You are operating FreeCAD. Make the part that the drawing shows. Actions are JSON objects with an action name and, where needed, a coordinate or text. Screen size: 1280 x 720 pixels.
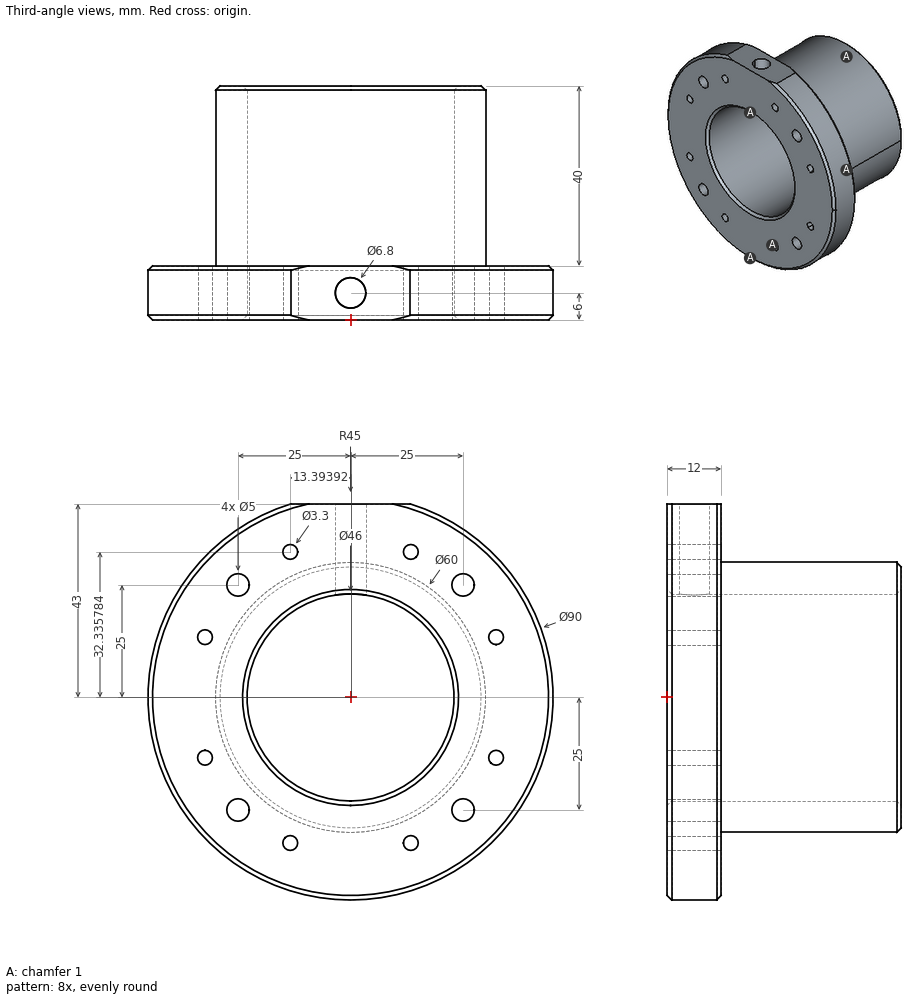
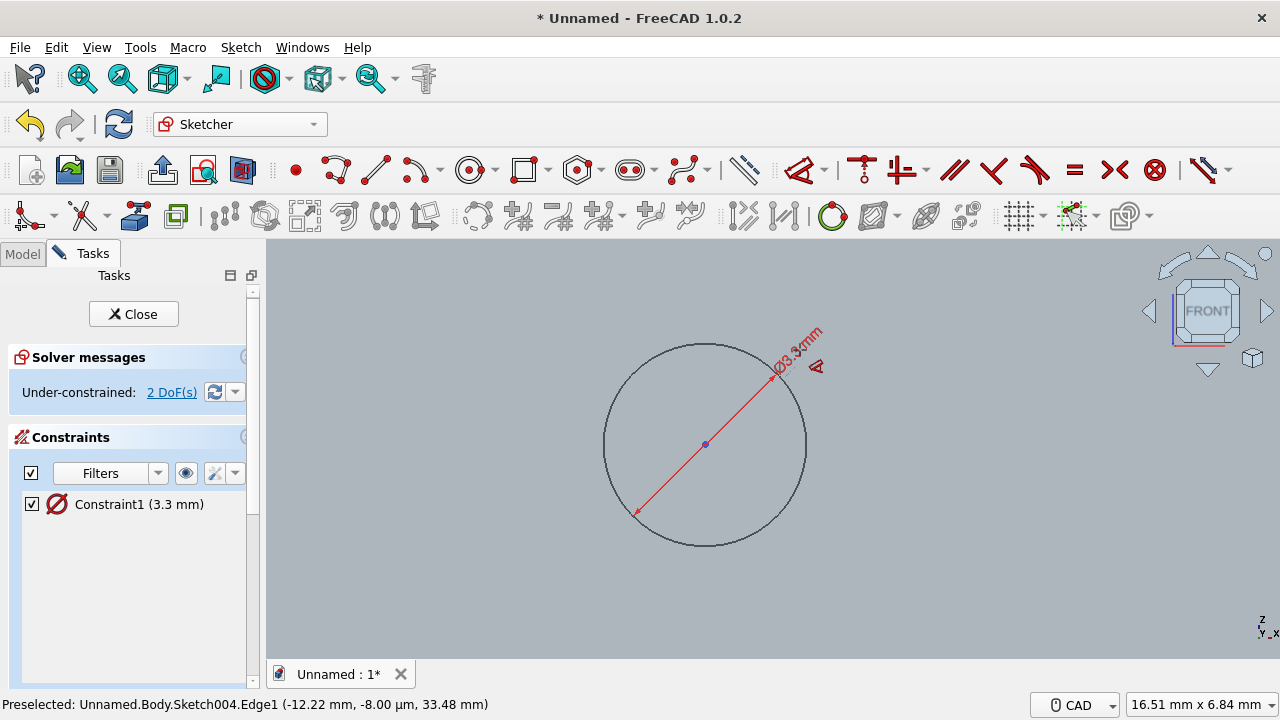
{"action": "left_click", "coordinate": [705, 445]}
{"action": "left_click", "coordinate": [910, 411]}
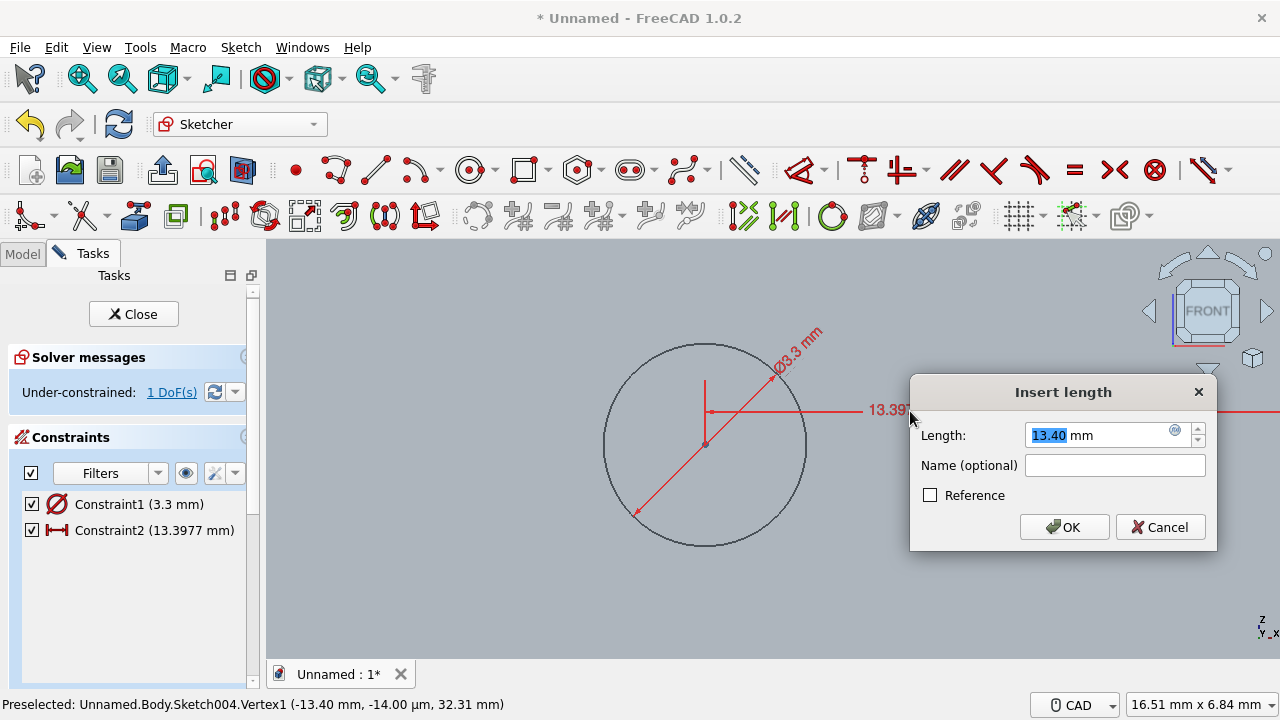
{"action": "type", "text": "13.39392"}
{"action": "key", "text": "Return"}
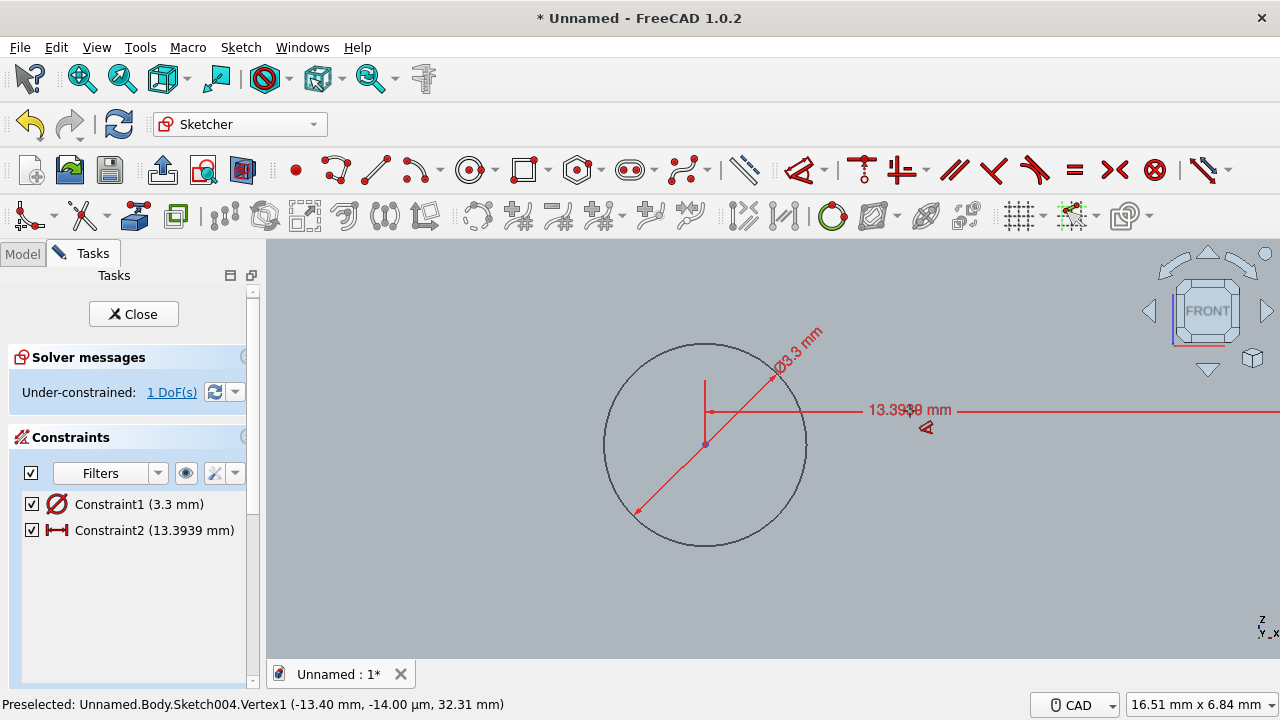
{"action": "left_click", "coordinate": [705, 445]}
{"action": "left_click", "coordinate": [671, 495]}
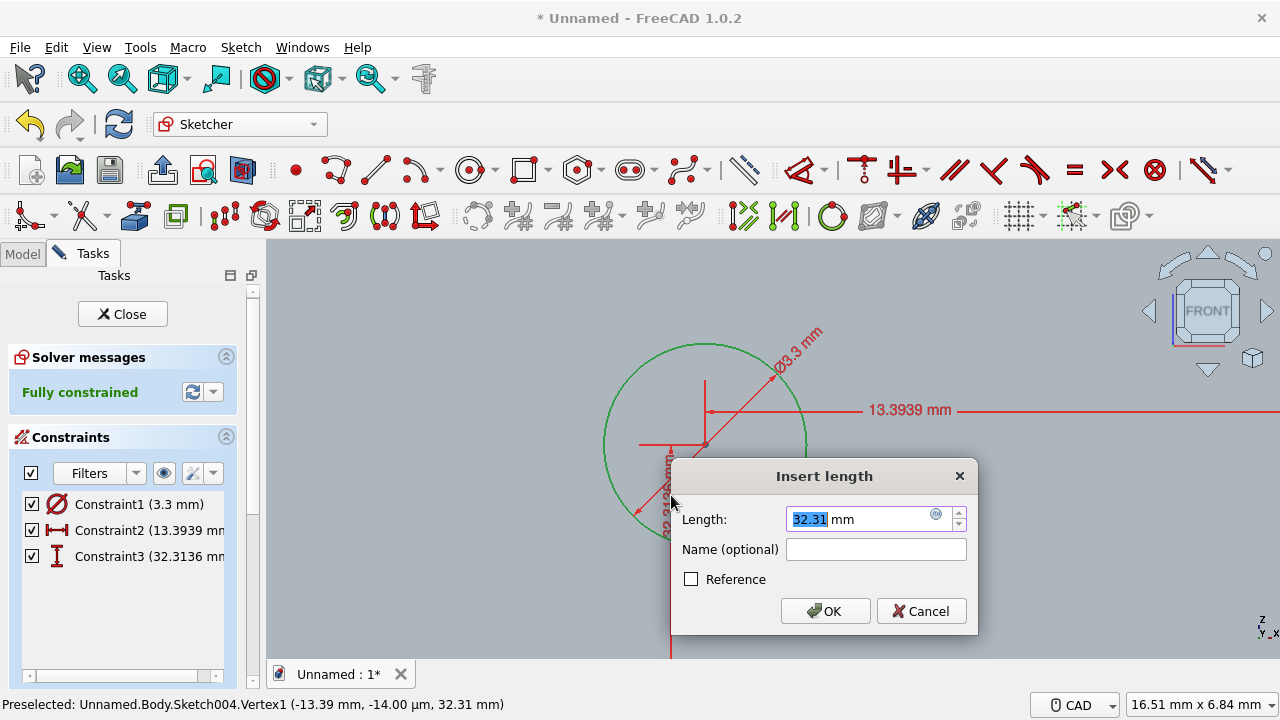
{"action": "type", "text": "32.335784"}
{"action": "key", "text": "Return"}
{"action": "key", "text": "Escape"}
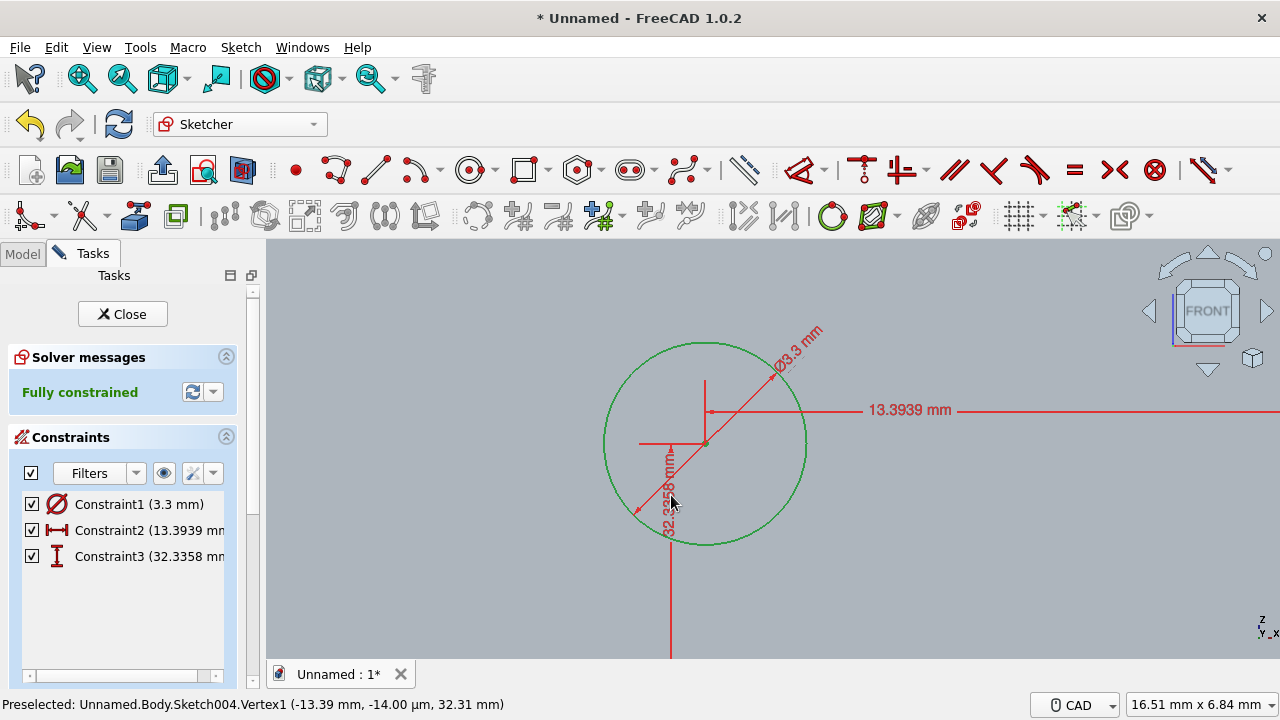
{"action": "left_click", "coordinate": [123, 314]}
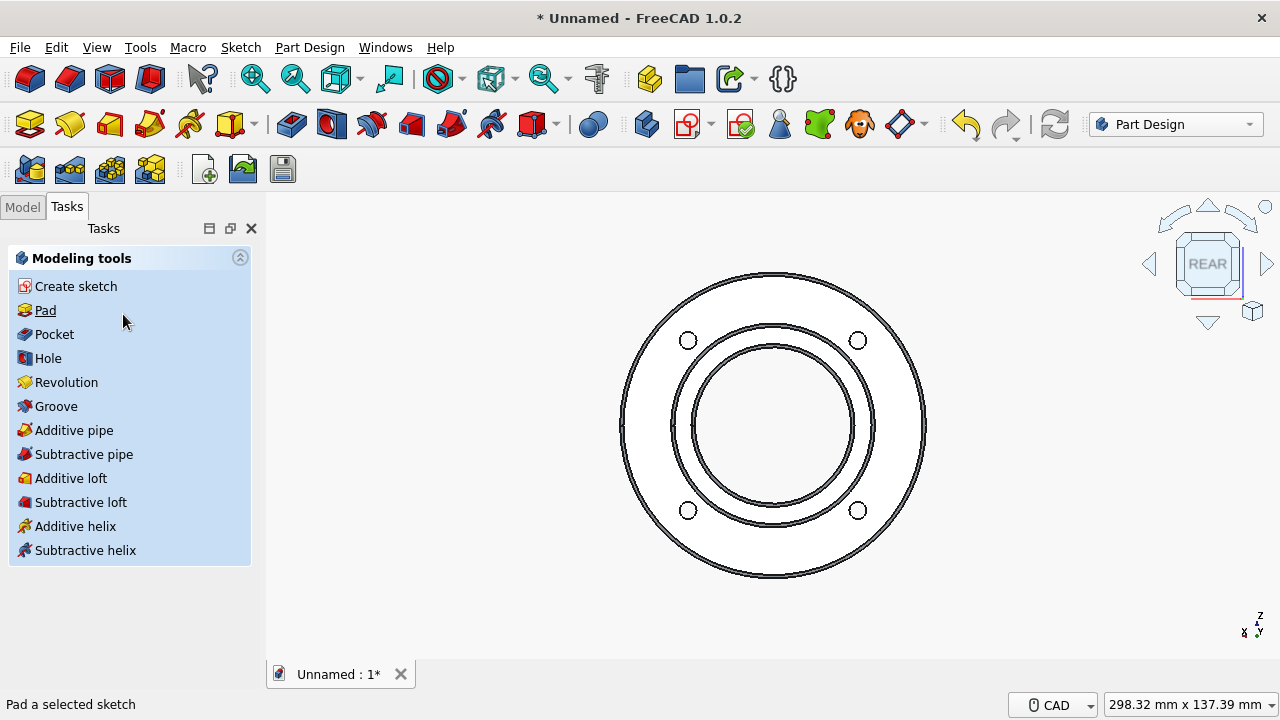
{"action": "left_click", "coordinate": [292, 124]}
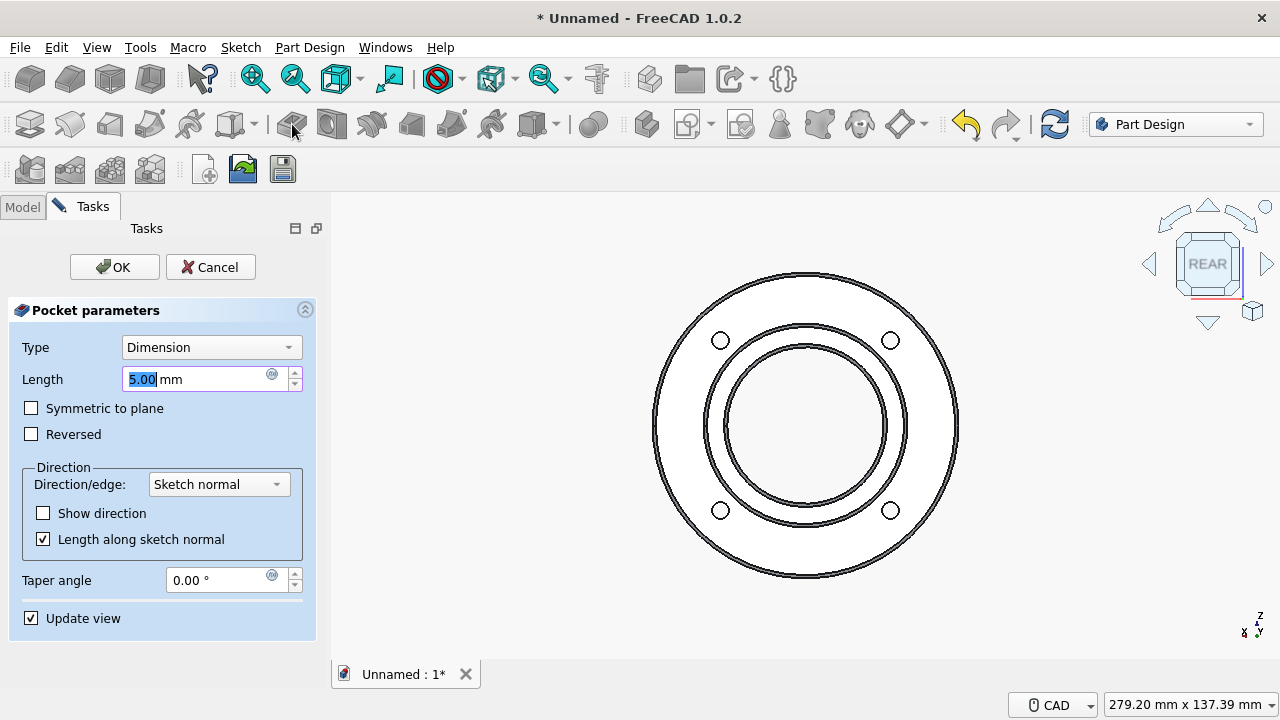
{"action": "left_click", "coordinate": [212, 348]}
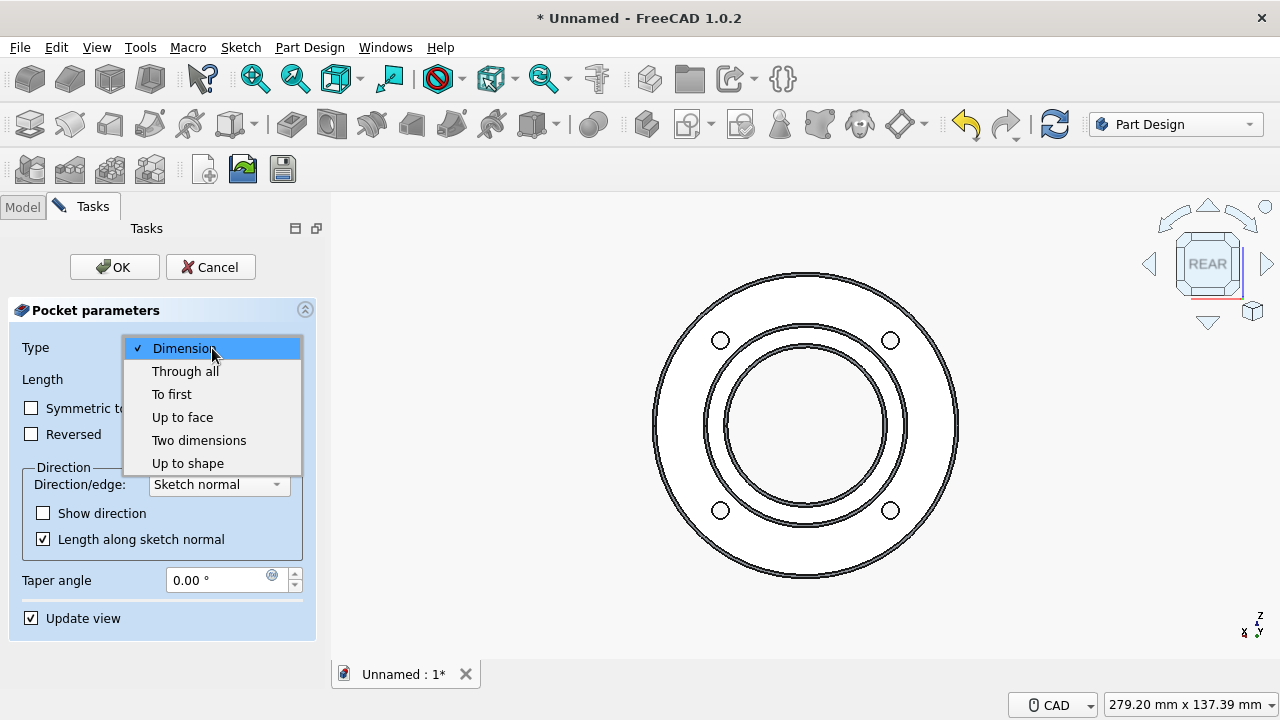
{"action": "left_click", "coordinate": [212, 372]}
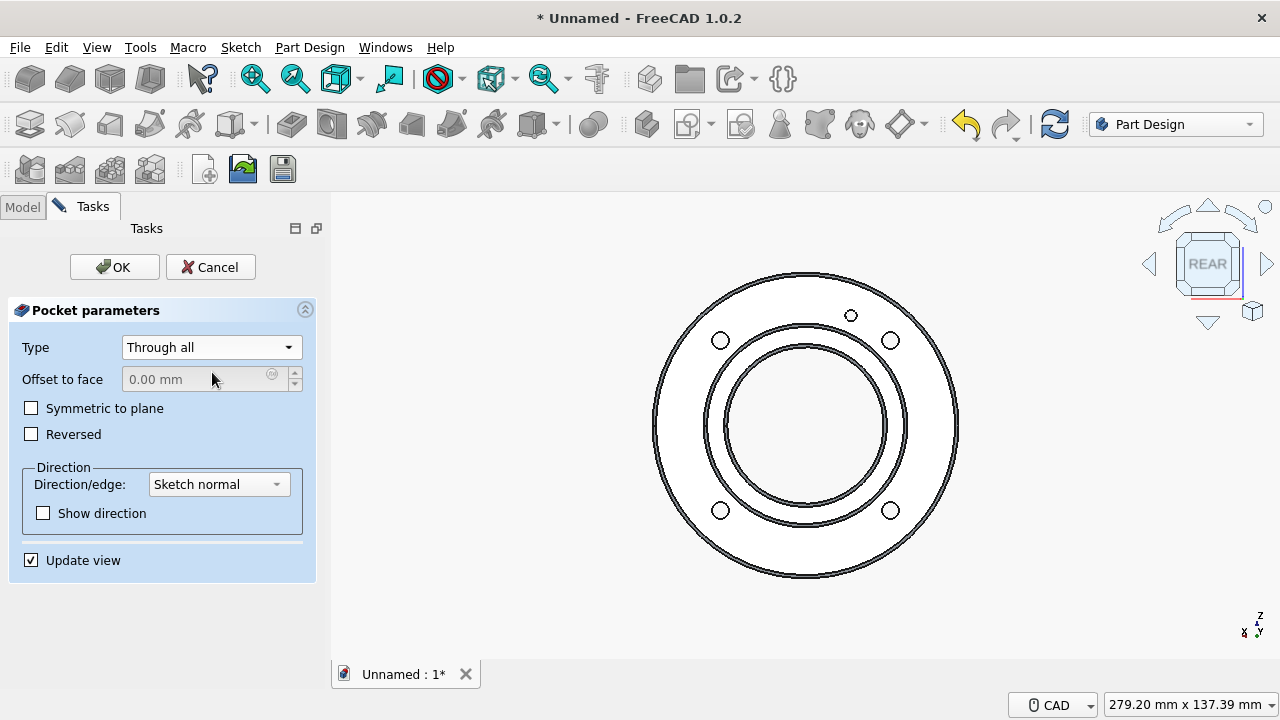
{"action": "left_click", "coordinate": [115, 267]}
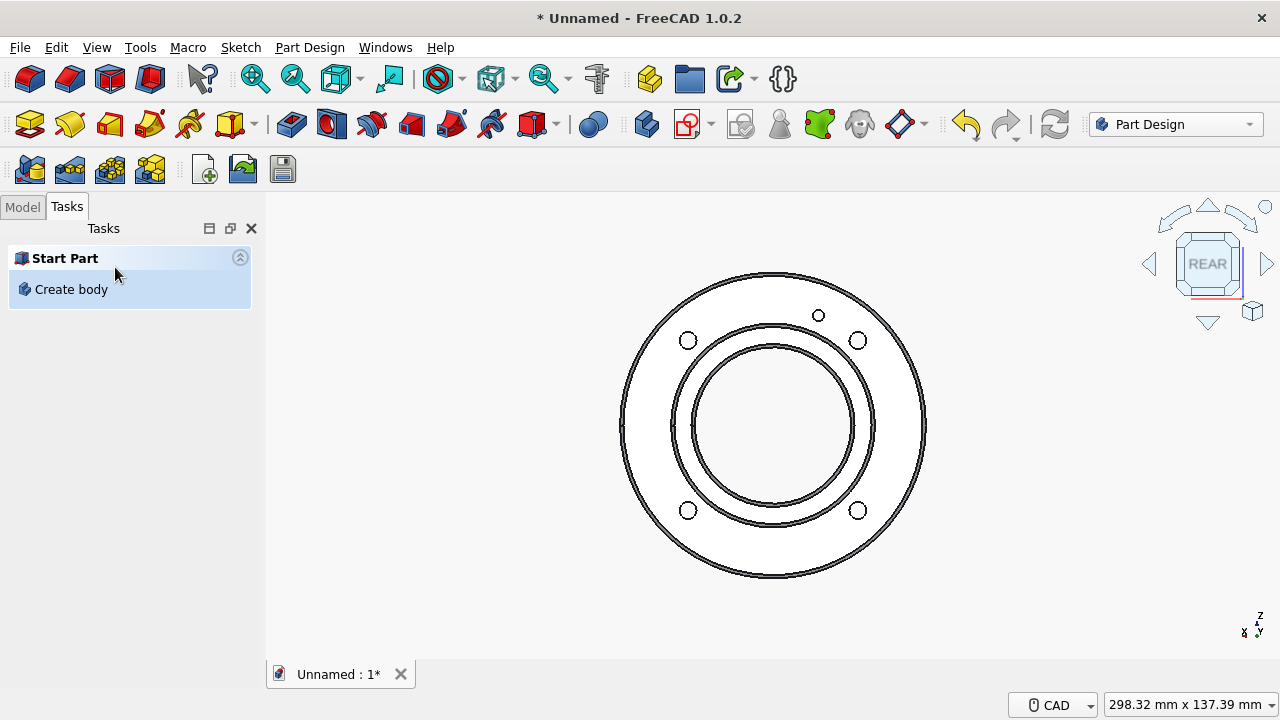
{"action": "left_click", "coordinate": [688, 124]}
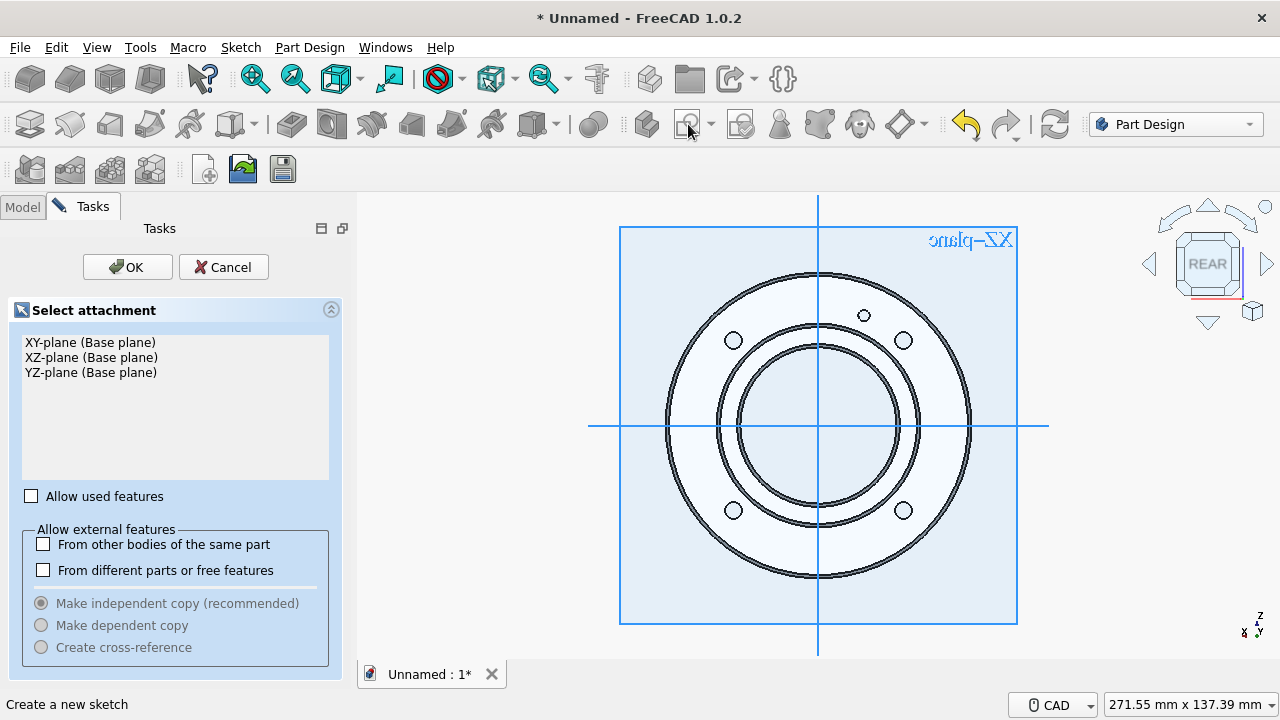
{"action": "left_click", "coordinate": [82, 358]}